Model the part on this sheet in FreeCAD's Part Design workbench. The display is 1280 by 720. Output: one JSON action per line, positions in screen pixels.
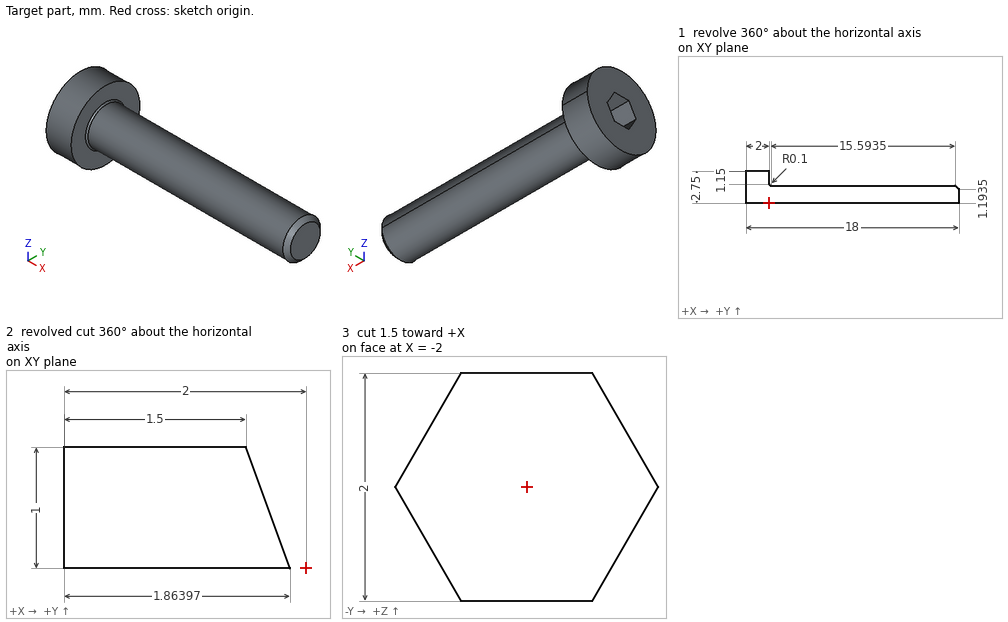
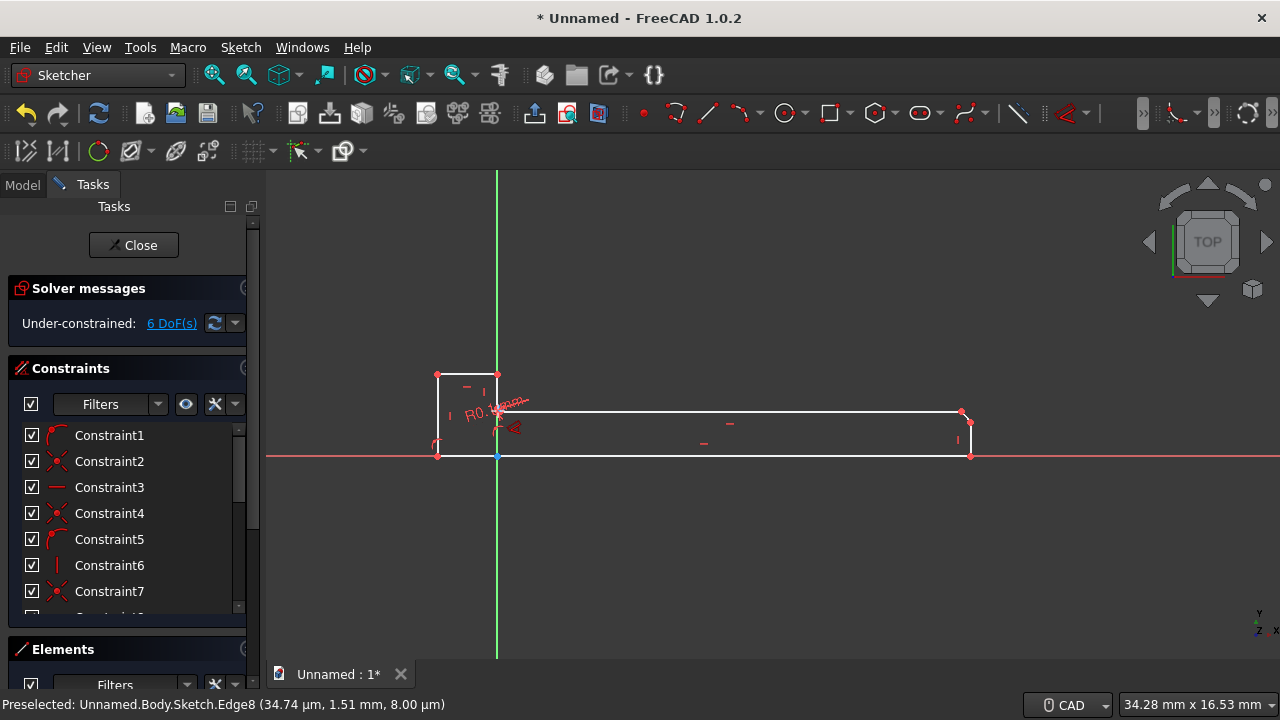
{"action": "left_click", "coordinate": [479, 374]}
{"action": "left_click", "coordinate": [468, 340]}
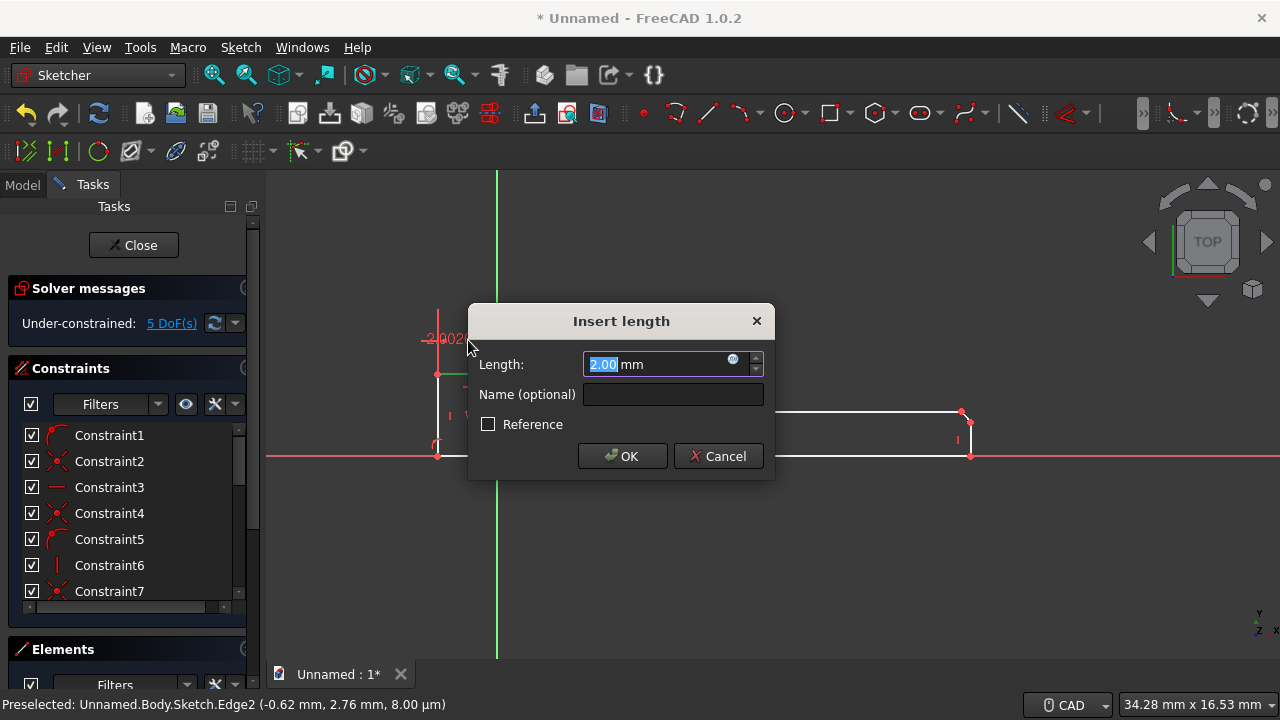
{"action": "type", "text": "2"}
{"action": "key", "text": "Return"}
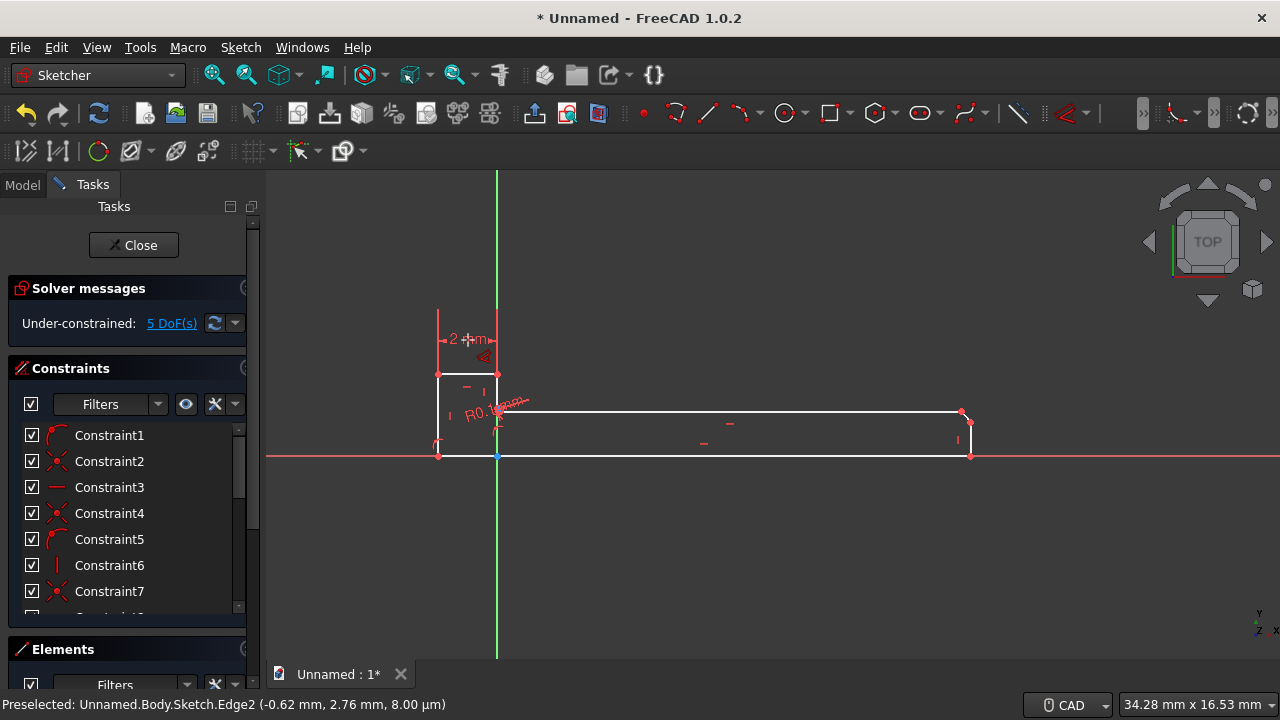
{"action": "left_click", "coordinate": [598, 456]}
{"action": "left_click", "coordinate": [704, 490]}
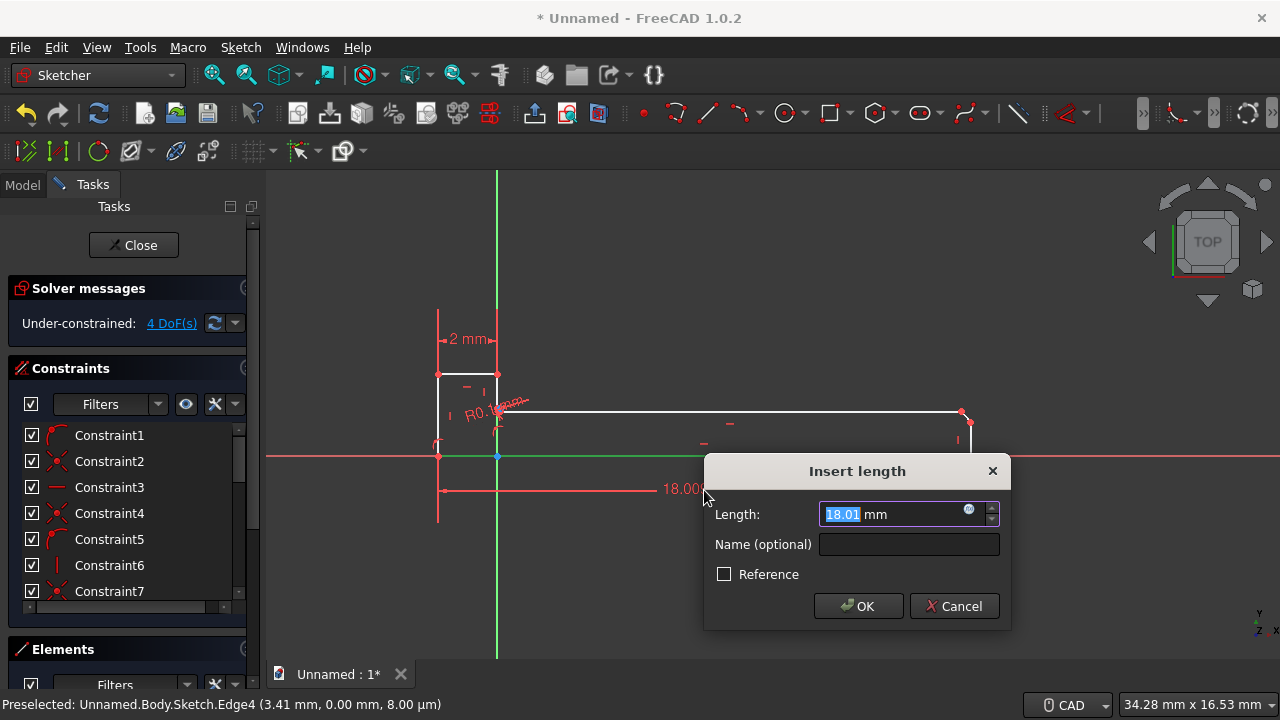
{"action": "type", "text": "18"}
{"action": "key", "text": "Return"}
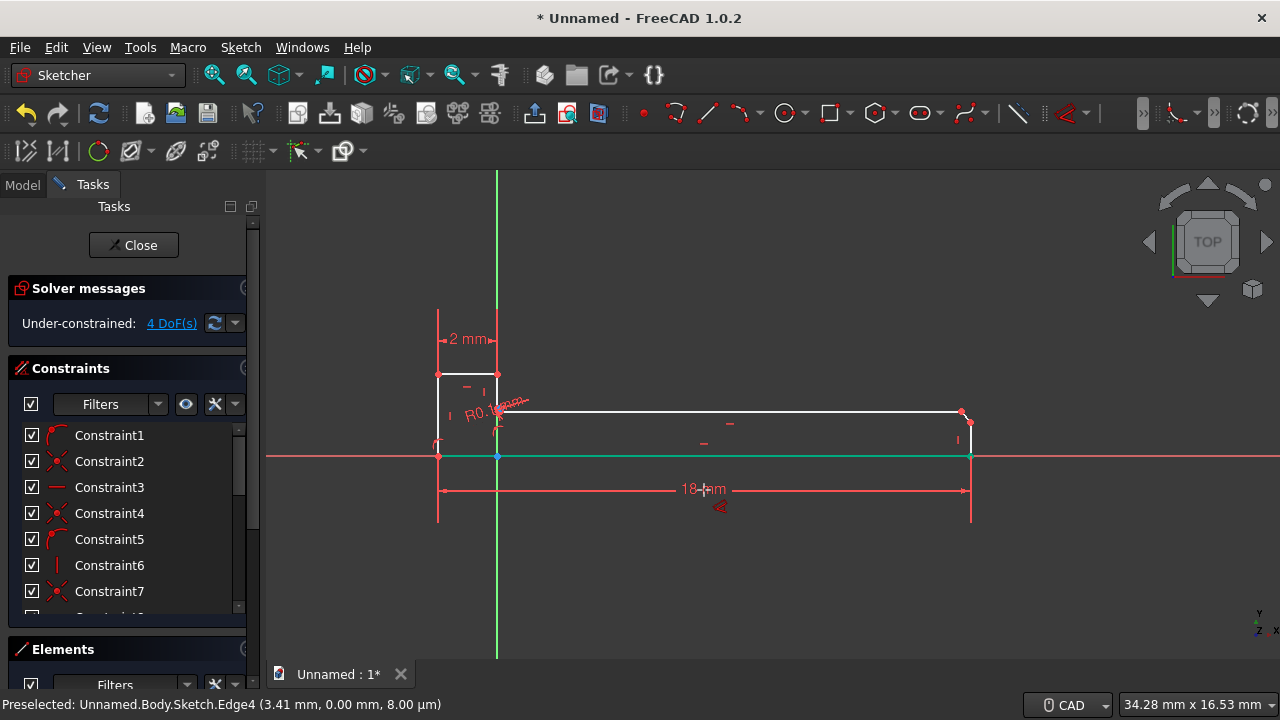
{"action": "scroll", "coordinate": [497, 398], "scroll_direction": "up", "scroll_amount": 2}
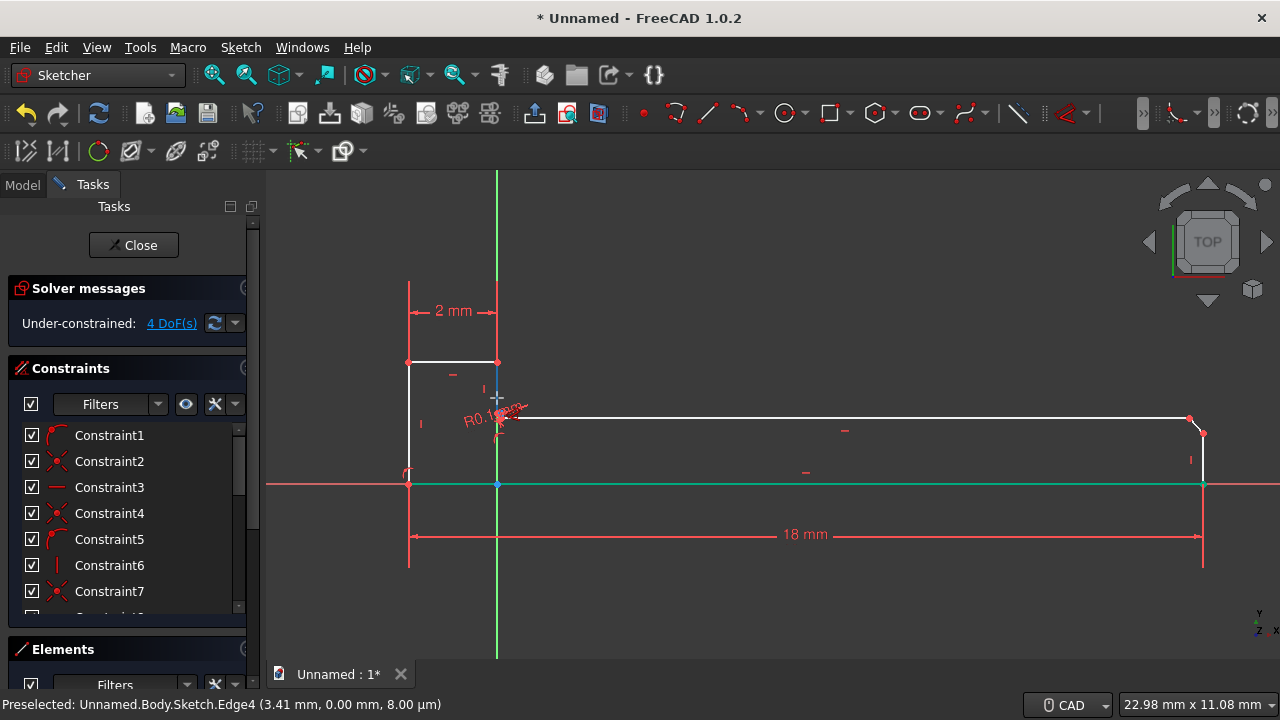
{"action": "left_click", "coordinate": [497, 398]}
{"action": "left_click", "coordinate": [463, 388]}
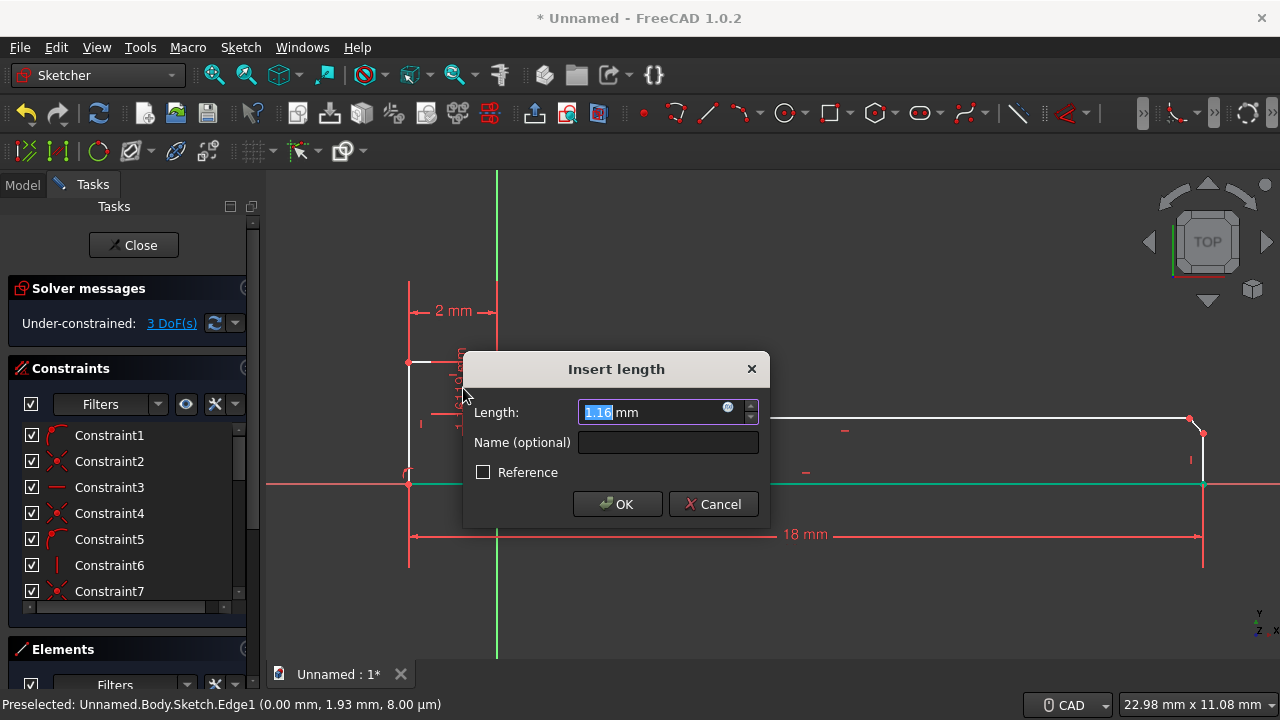
{"action": "type", "text": "1.15"}
{"action": "key", "text": "Return"}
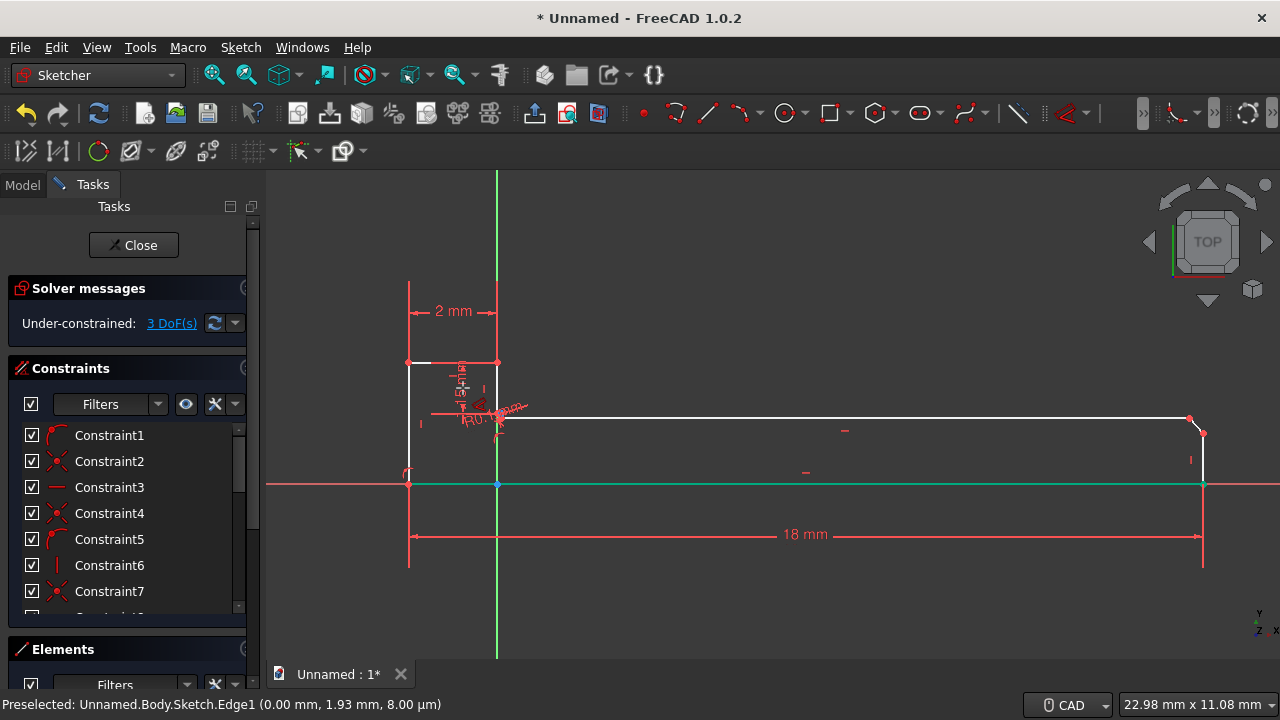
{"action": "left_click", "coordinate": [409, 399]}
{"action": "left_click", "coordinate": [375, 424]}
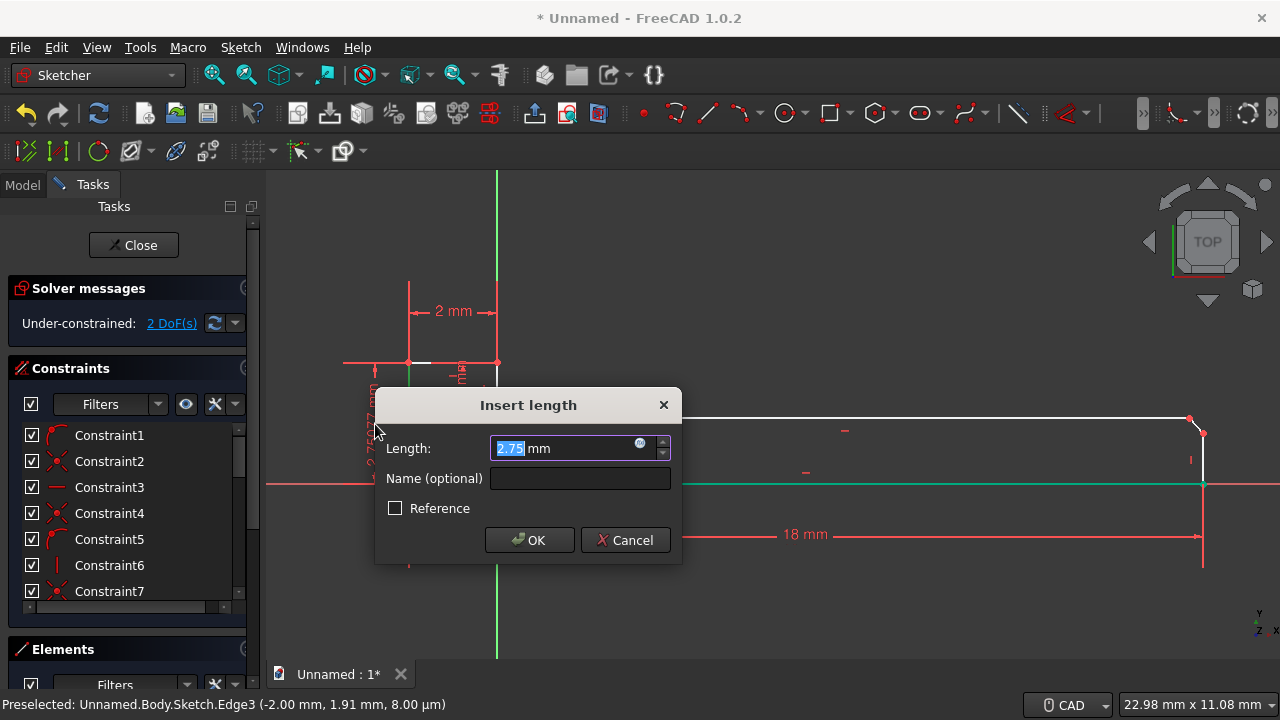
{"action": "type", "text": "2.75"}
{"action": "key", "text": "Return"}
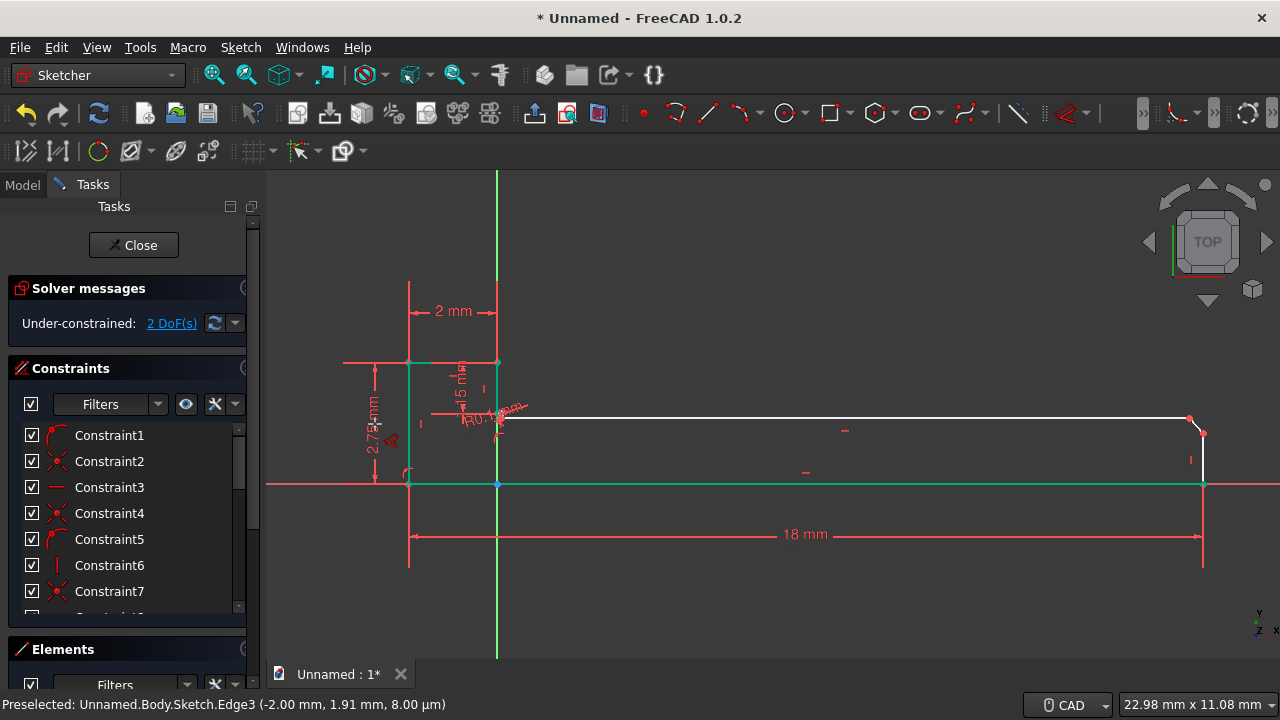
{"action": "scroll", "coordinate": [498, 396], "scroll_direction": "down", "scroll_amount": 2}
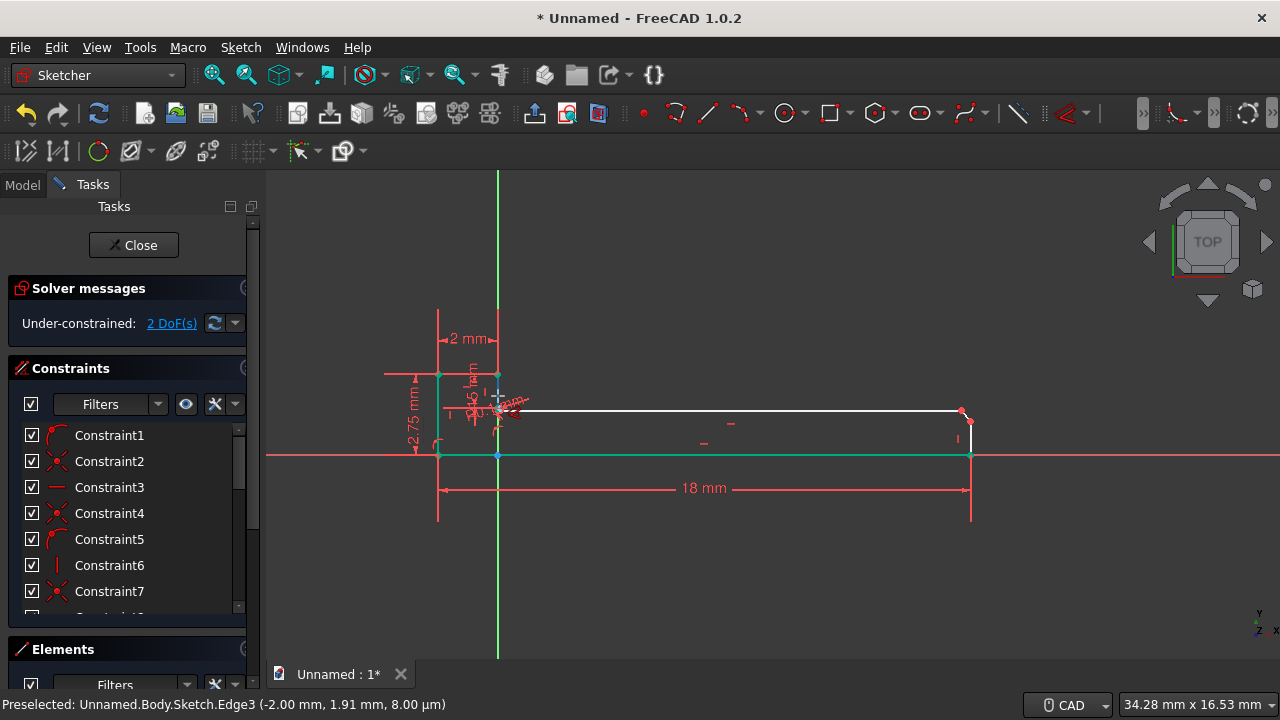
{"action": "scroll", "coordinate": [971, 445], "scroll_direction": "up", "scroll_amount": 2}